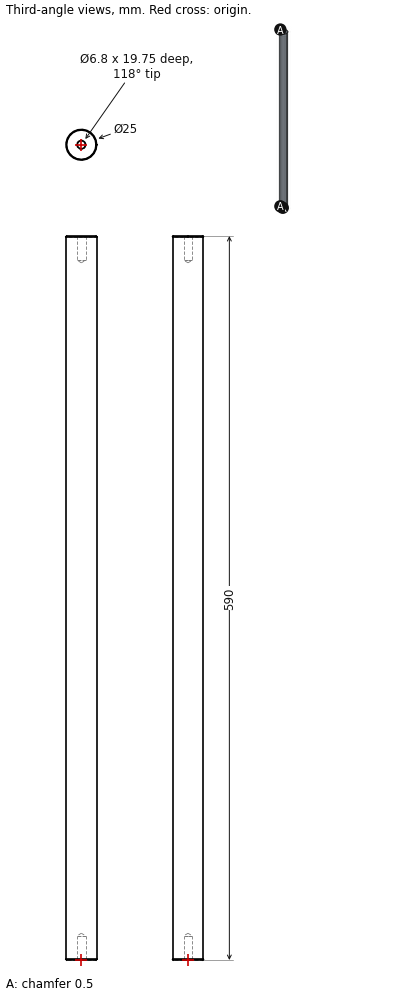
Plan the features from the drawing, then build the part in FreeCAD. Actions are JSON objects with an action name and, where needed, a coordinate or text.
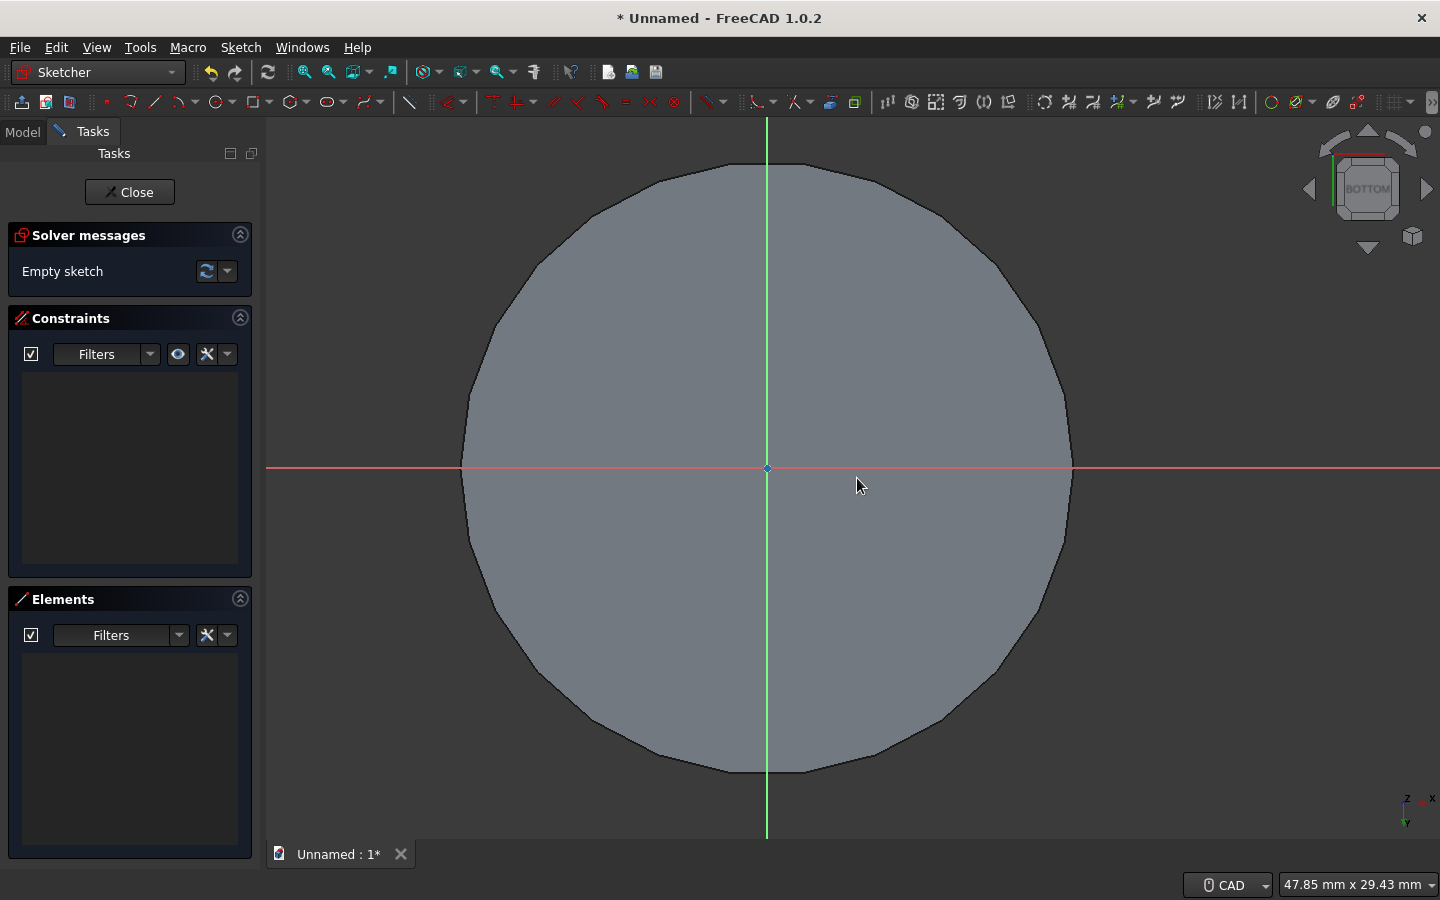
{"action": "scroll", "coordinate": [757, 463], "scroll_direction": "up", "scroll_amount": 5}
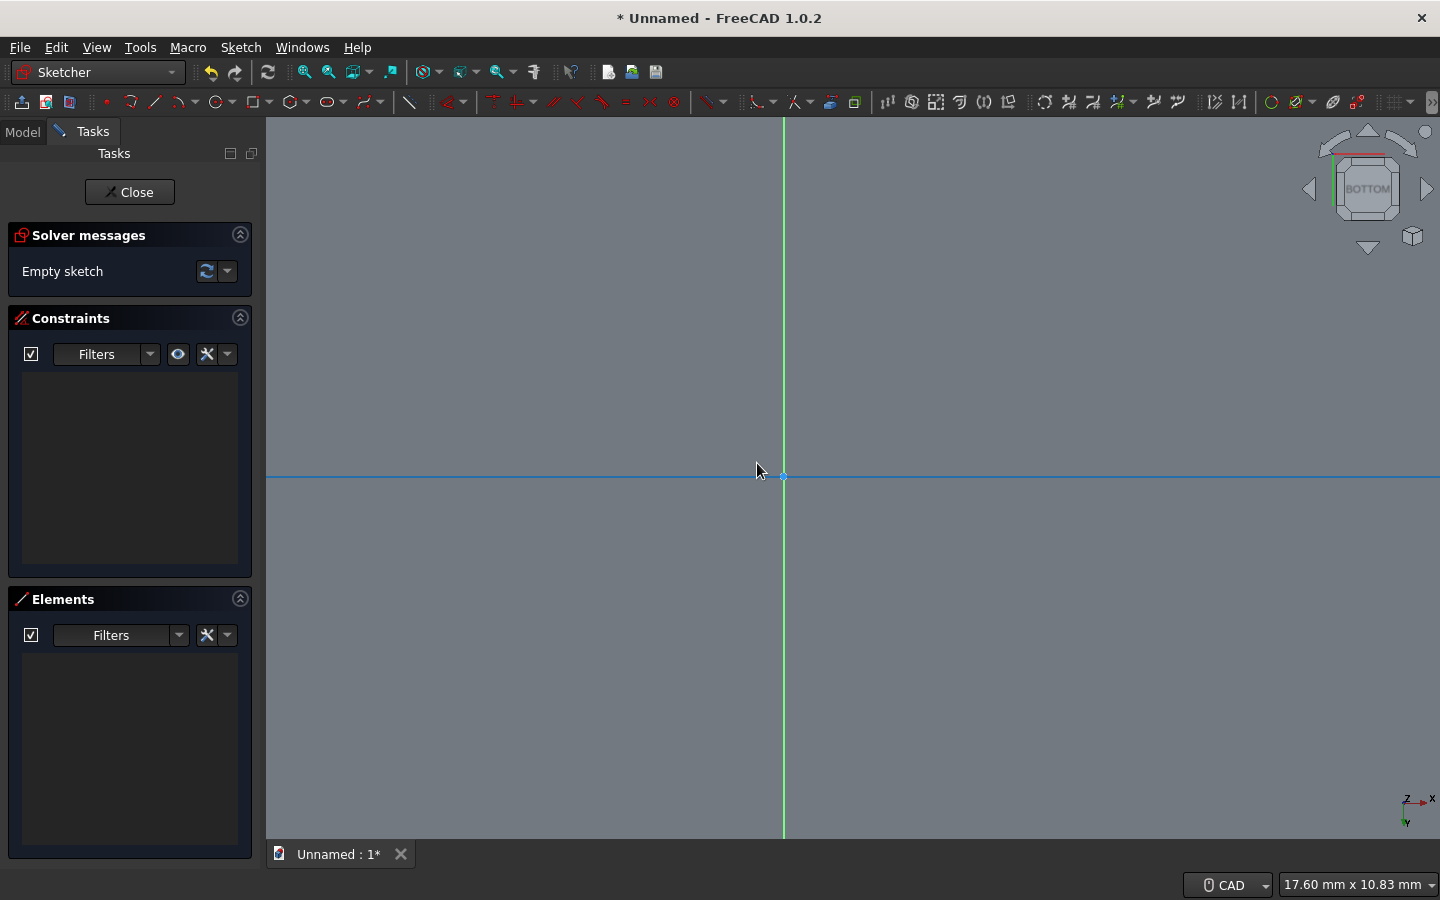
{"action": "key", "text": "g c"}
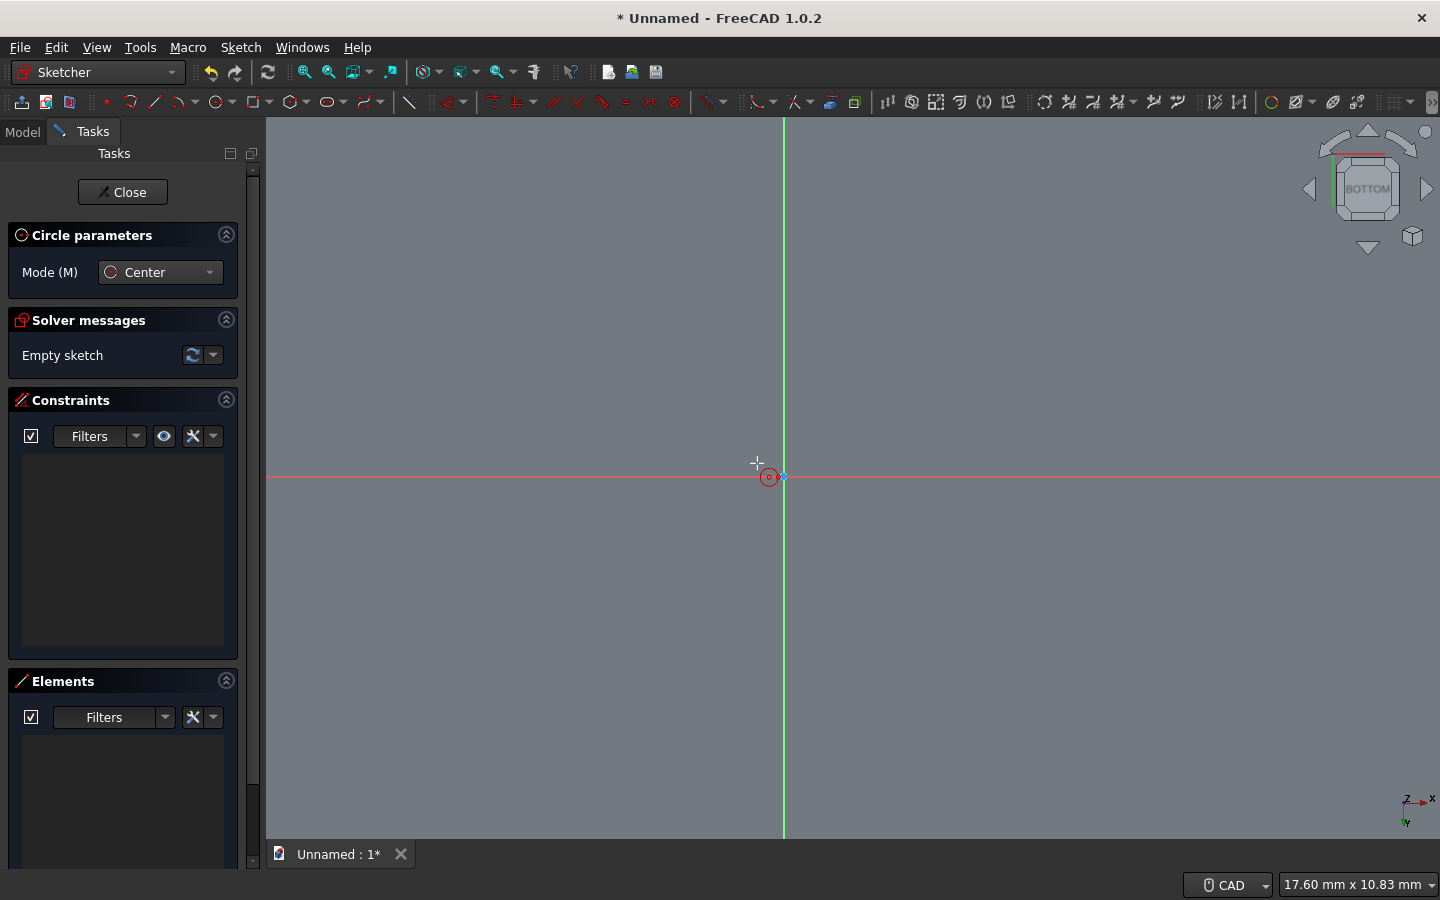
{"action": "left_click", "coordinate": [784, 477]}
{"action": "mouse_move", "coordinate": [944, 317]}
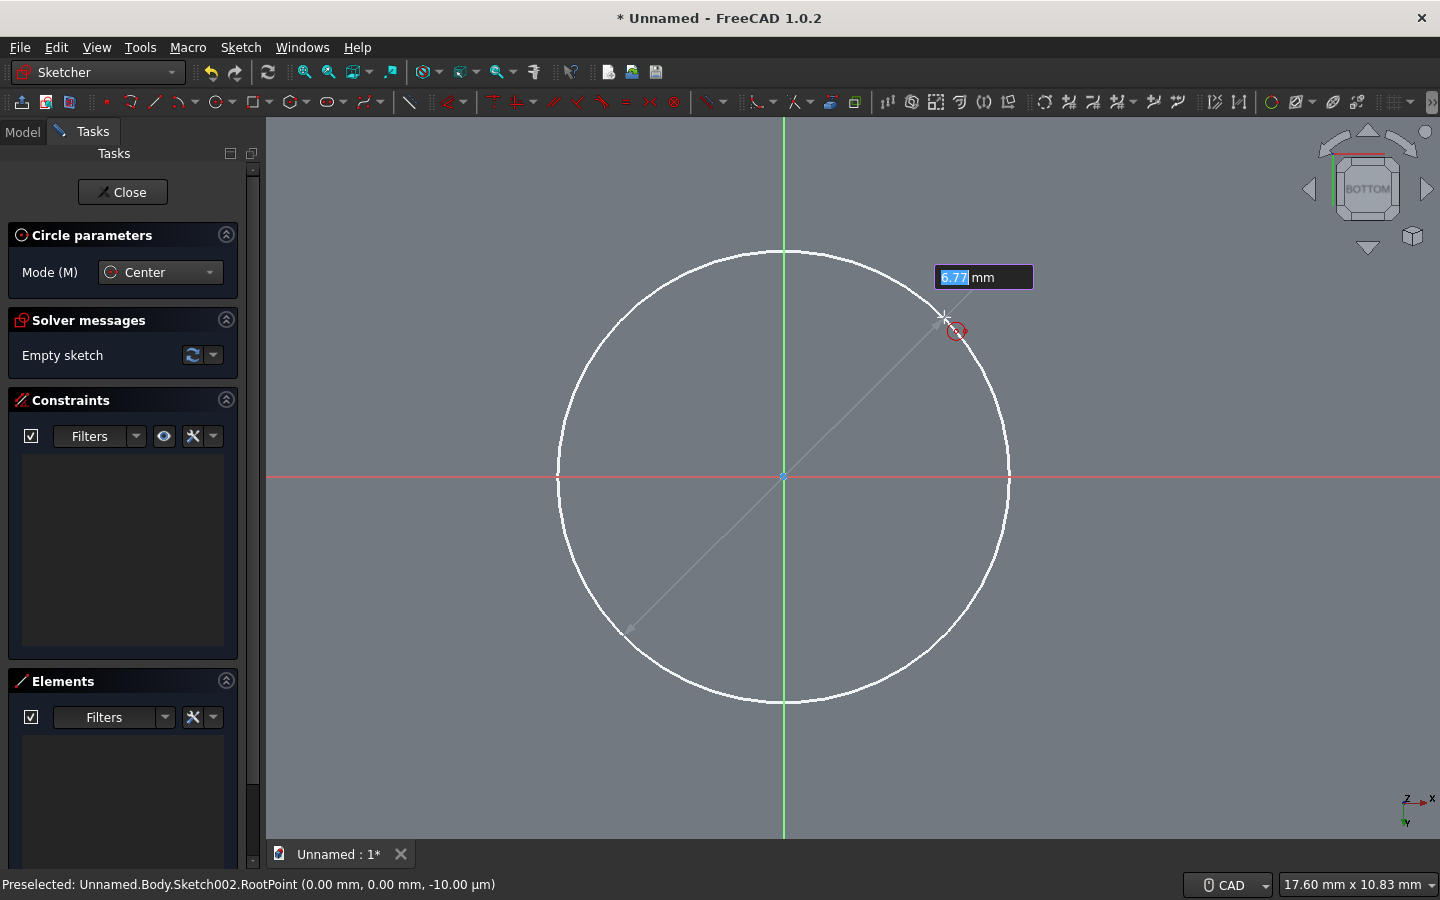
{"action": "type", "text": "6.8"}
{"action": "key", "text": "Return"}
{"action": "key", "text": "Escape"}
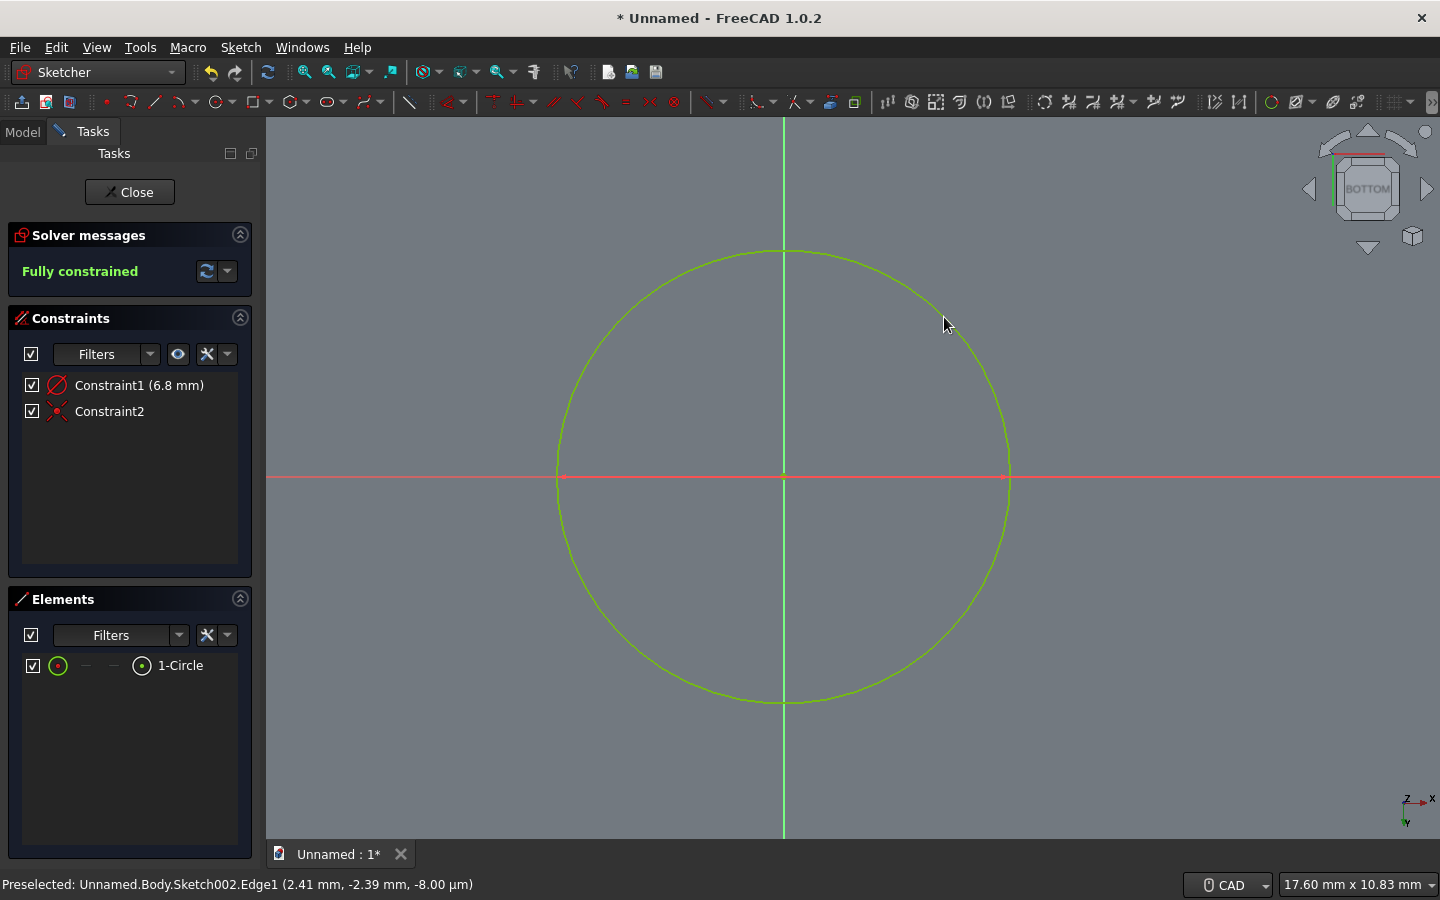
{"action": "left_click", "coordinate": [130, 192]}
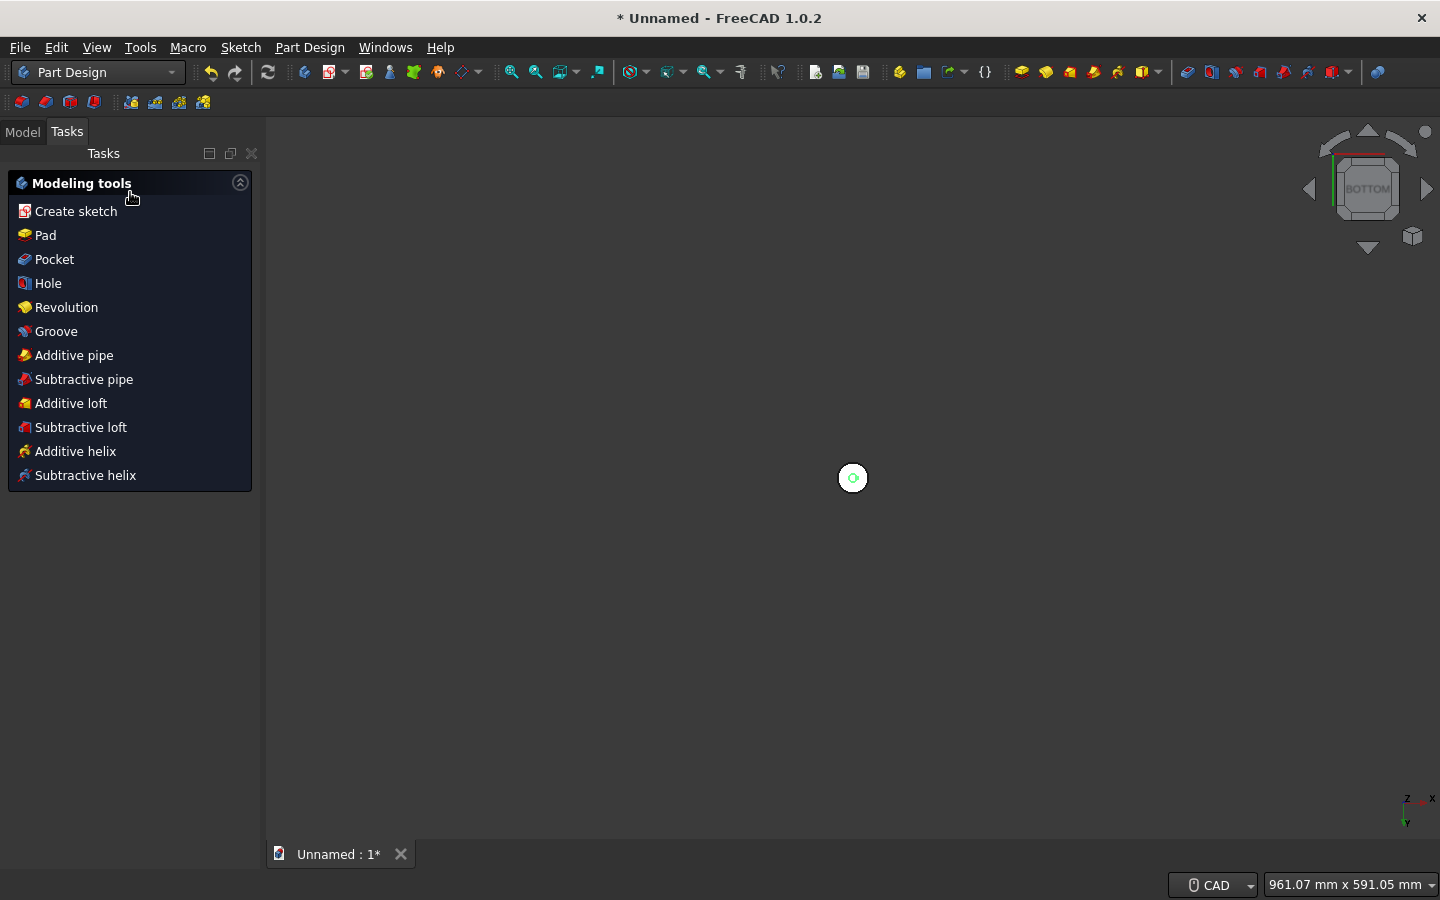
{"action": "left_click", "coordinate": [1212, 72]}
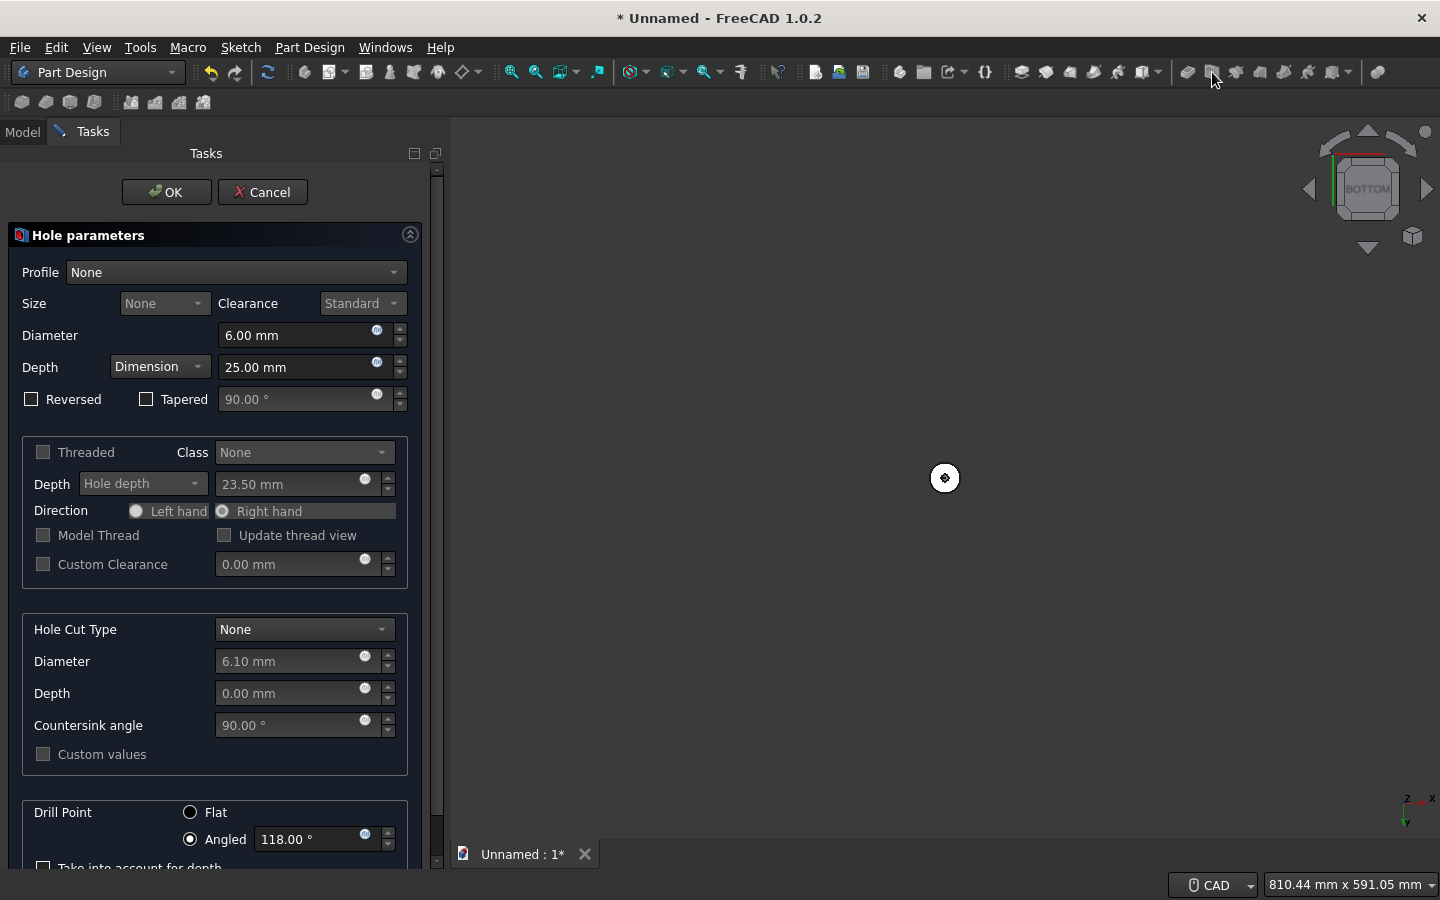
{"action": "triple_click", "coordinate": [305, 335]}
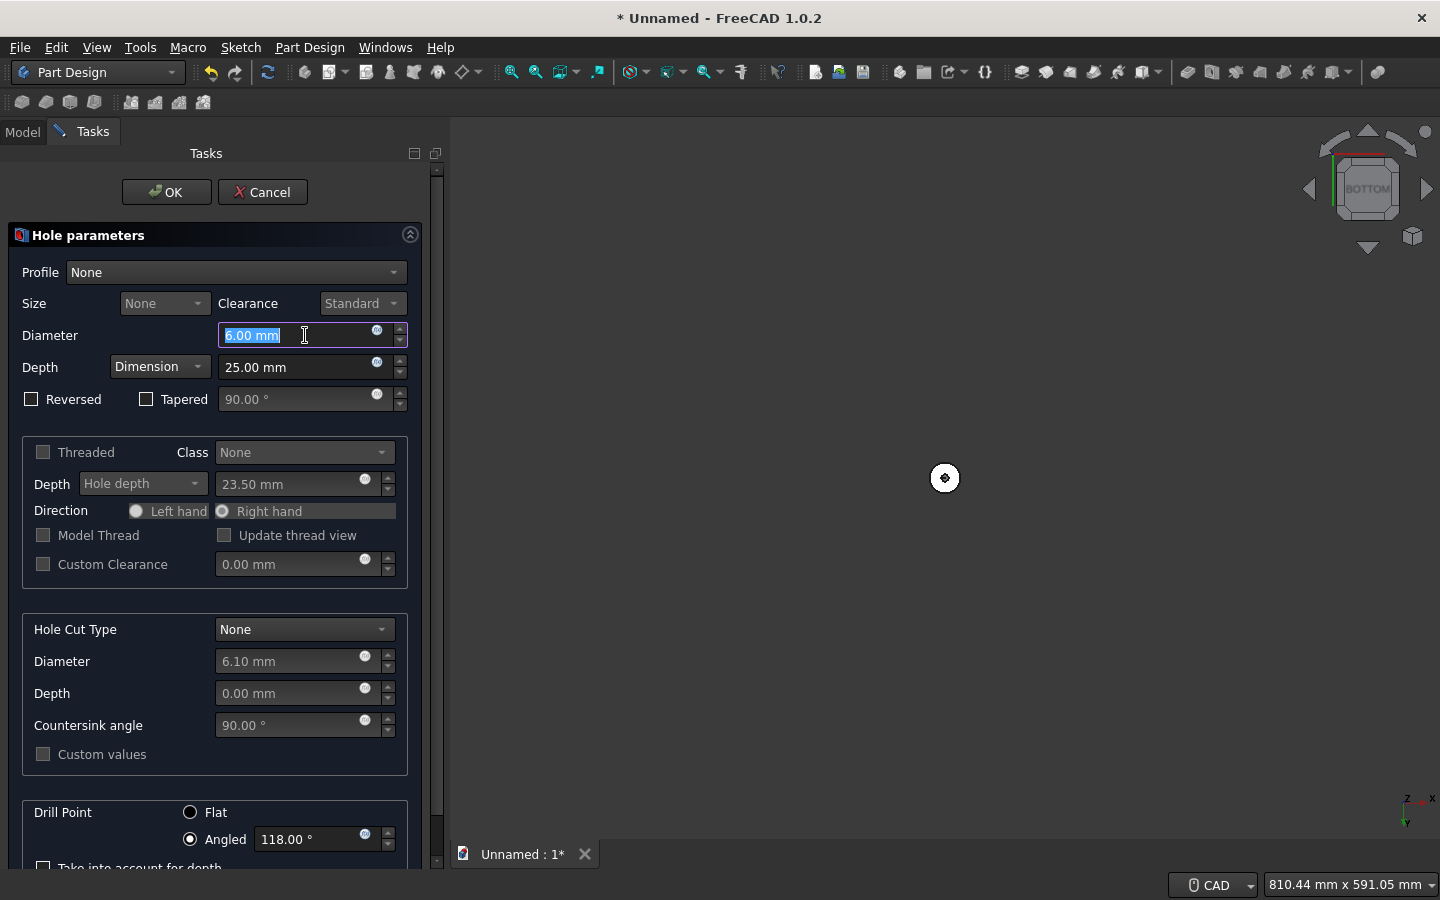
{"action": "type", "text": "6.8"}
{"action": "key", "text": "Tab"}